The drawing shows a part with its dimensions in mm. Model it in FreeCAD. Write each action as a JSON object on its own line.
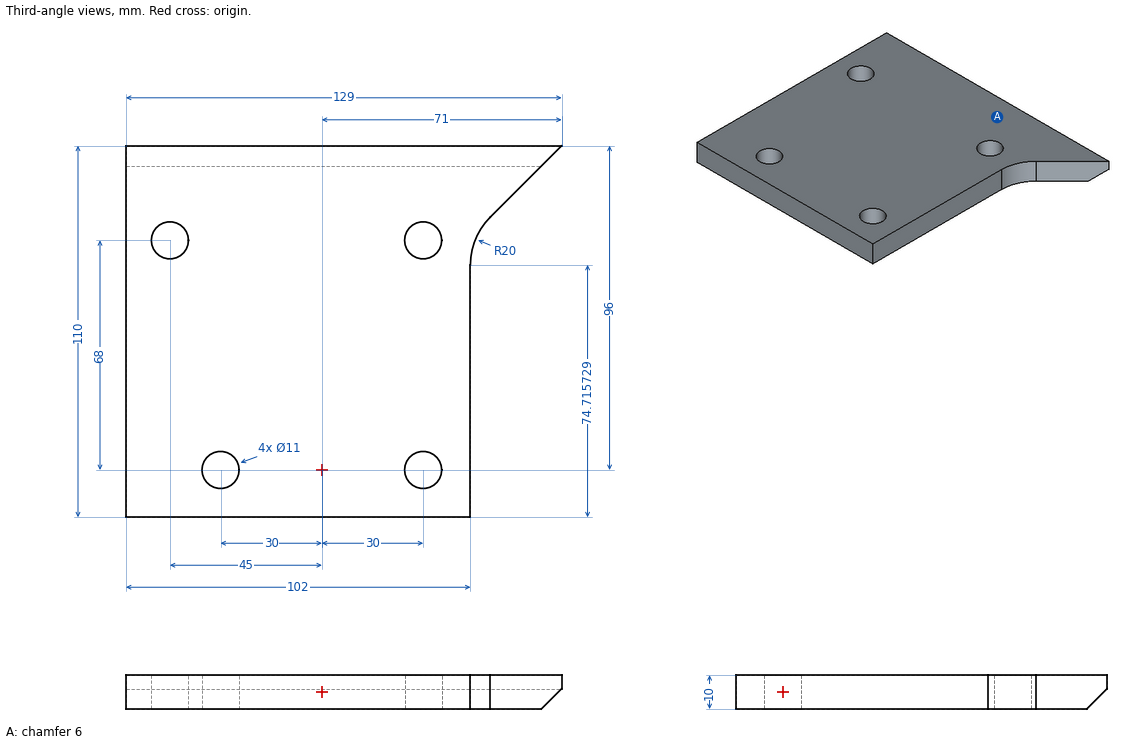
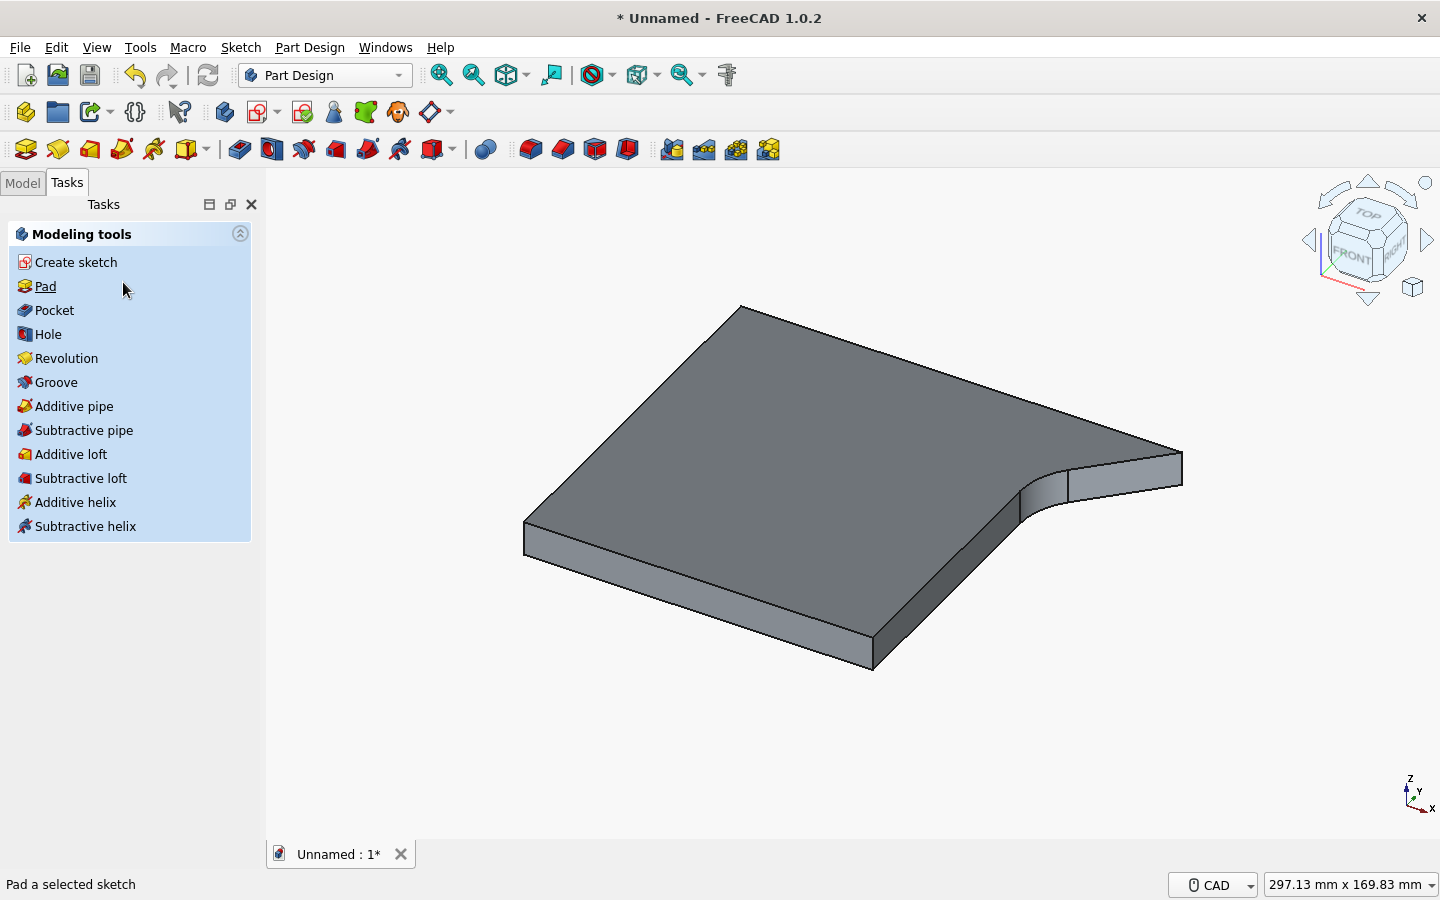
{"action": "left_click", "coordinate": [240, 150]}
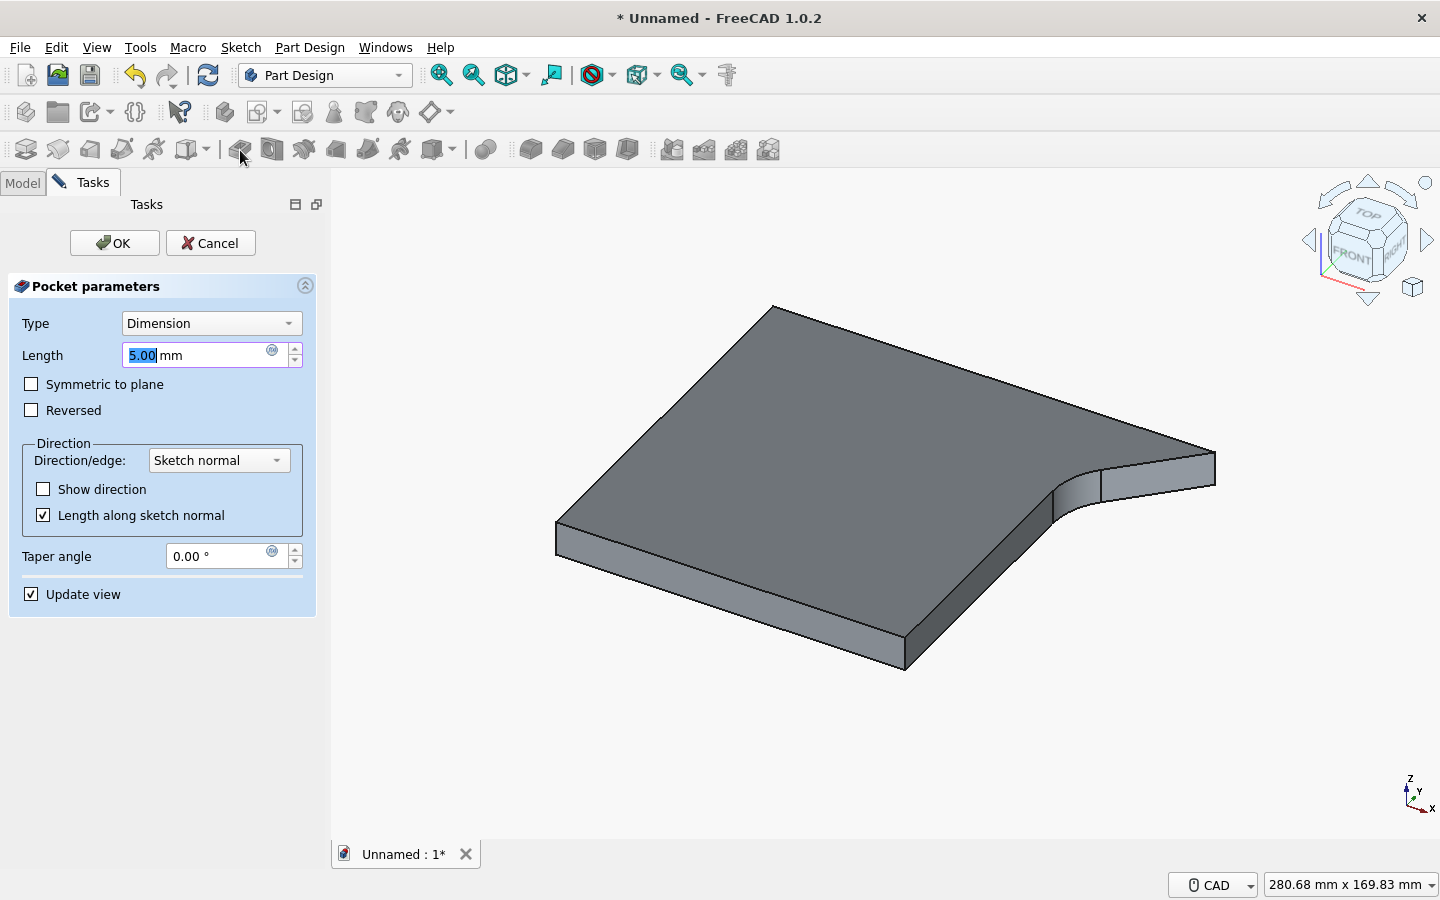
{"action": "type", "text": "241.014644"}
{"action": "key", "text": "Tab"}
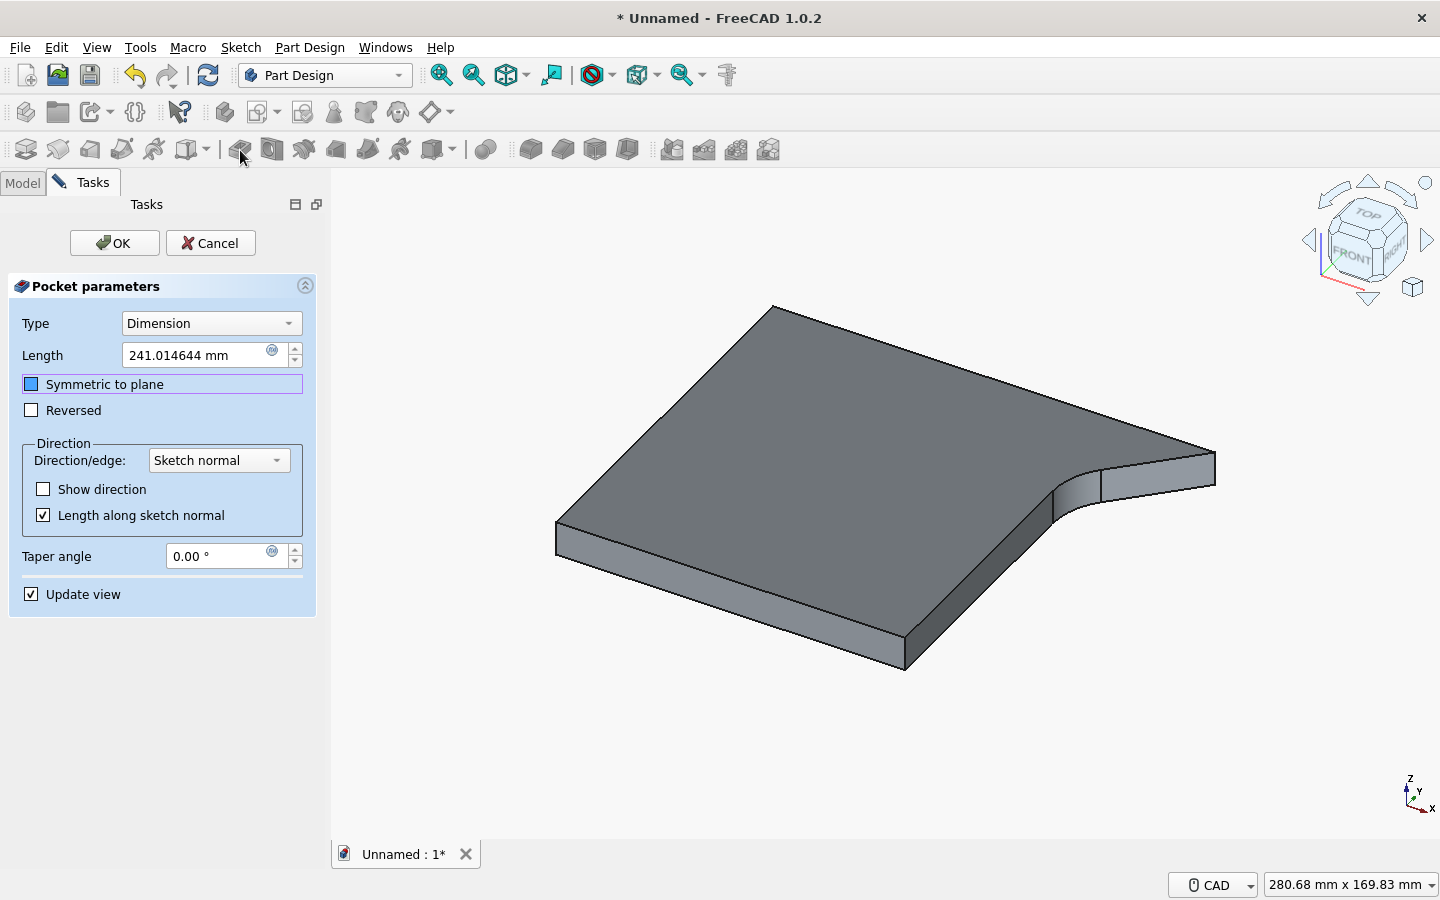
{"action": "left_click", "coordinate": [30, 384]}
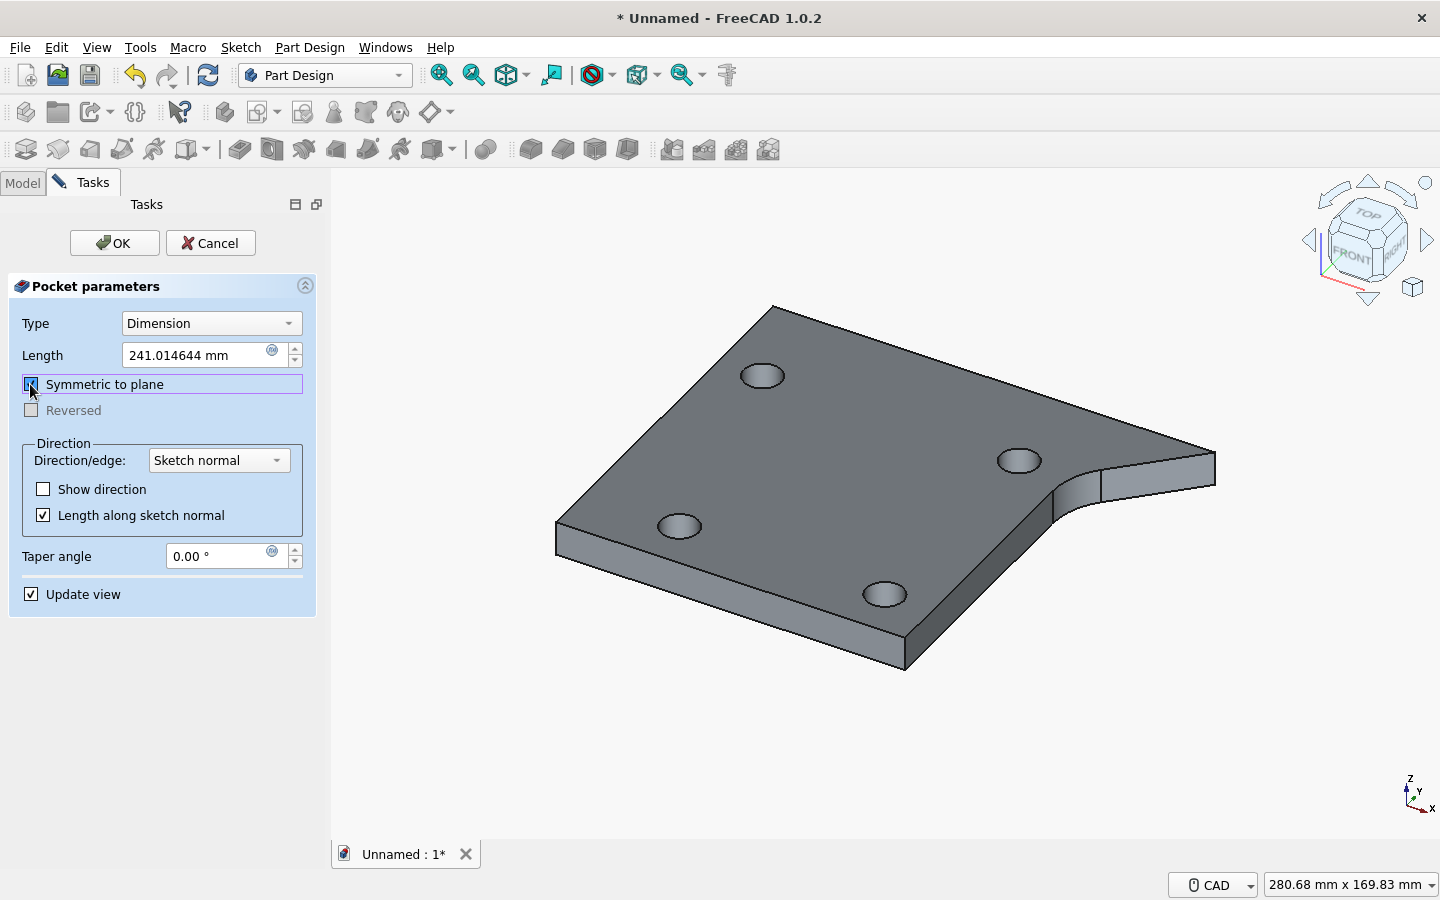
{"action": "left_click", "coordinate": [115, 243]}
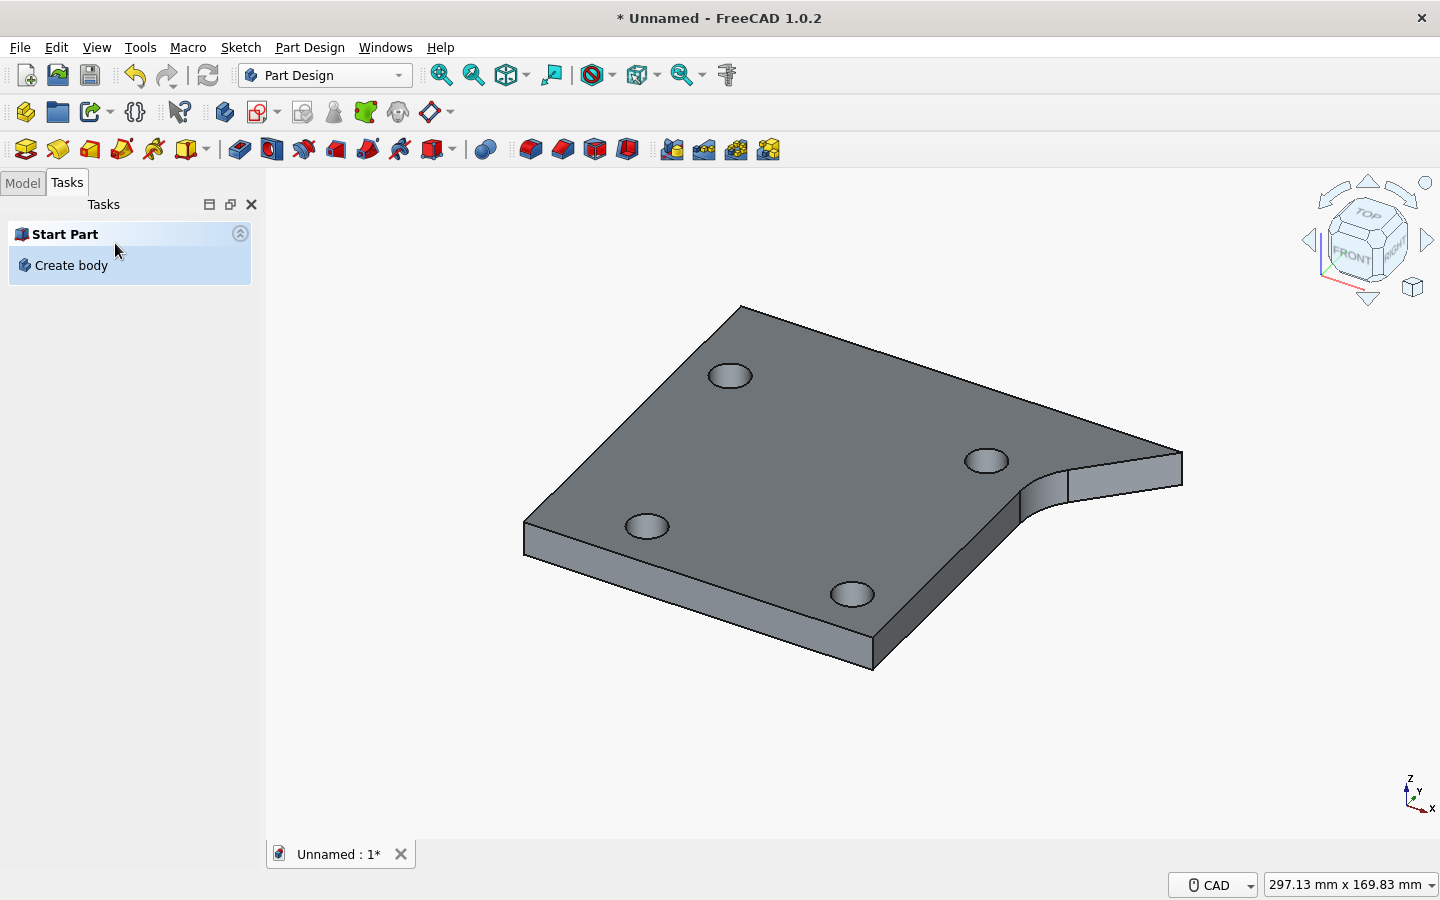
{"action": "key", "text": "0"}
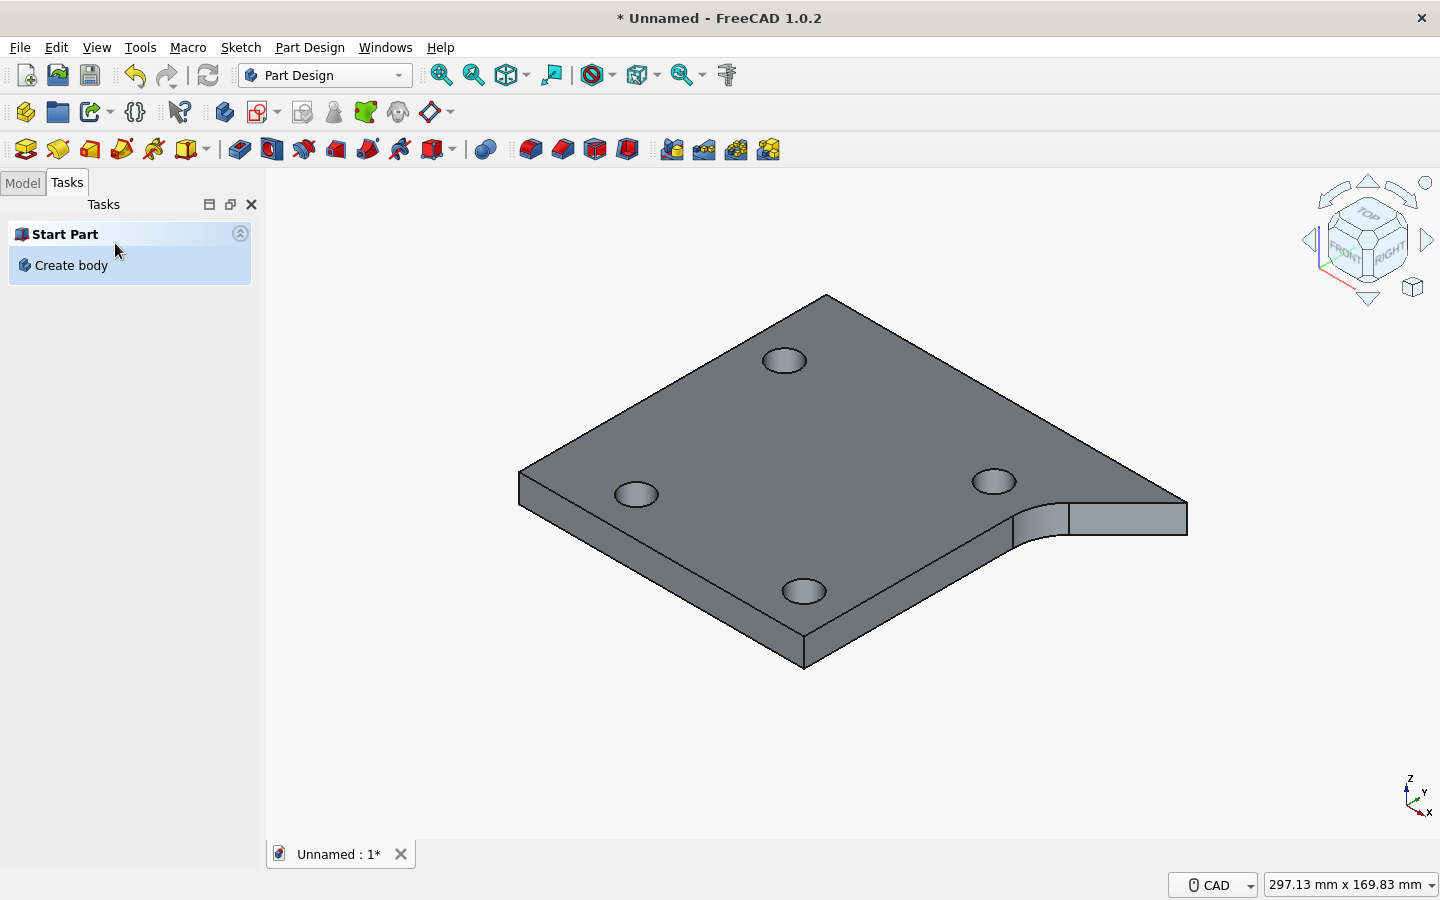
{"action": "key", "text": "2"}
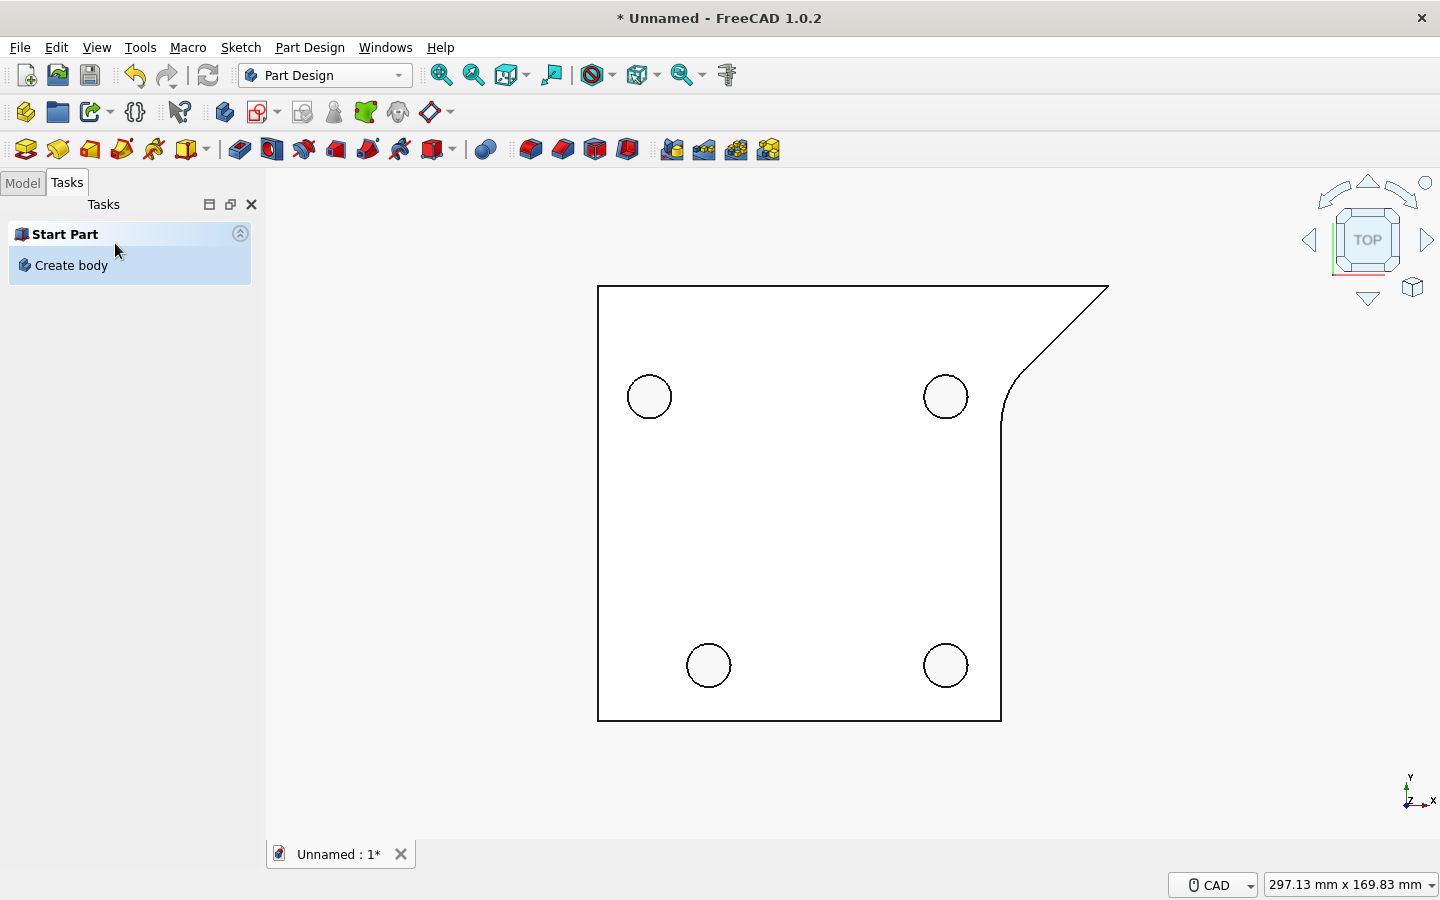
{"action": "key", "text": "1"}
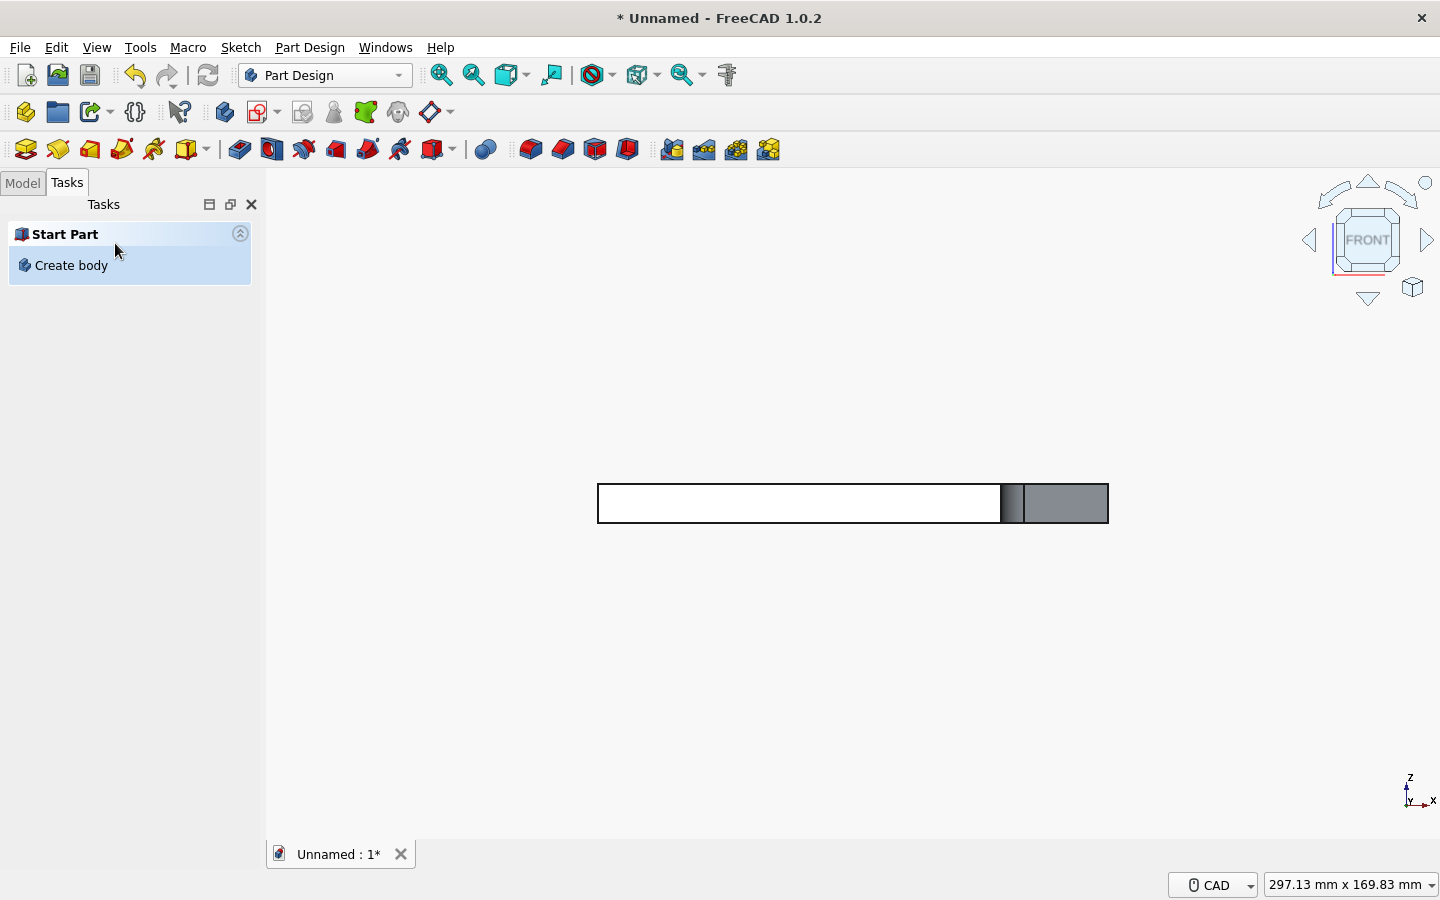
{"action": "key", "text": "v f"}